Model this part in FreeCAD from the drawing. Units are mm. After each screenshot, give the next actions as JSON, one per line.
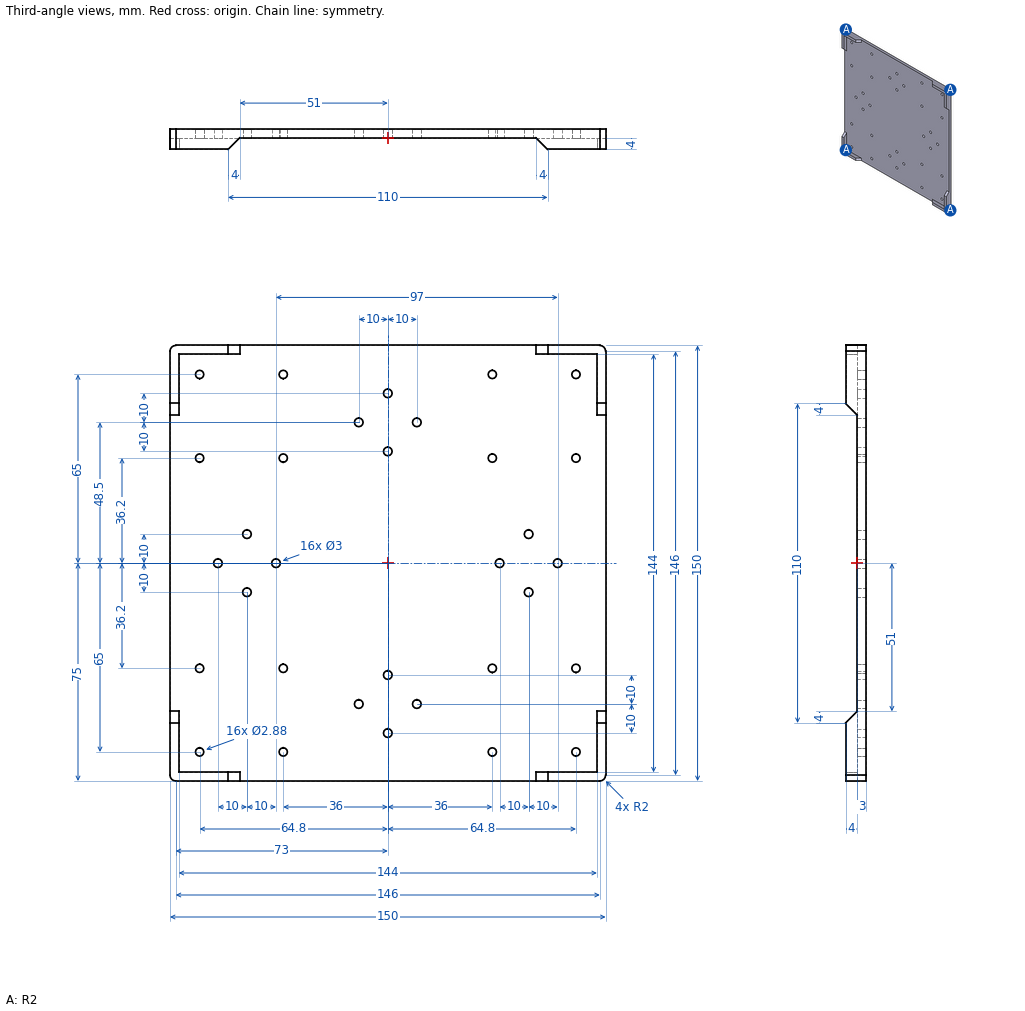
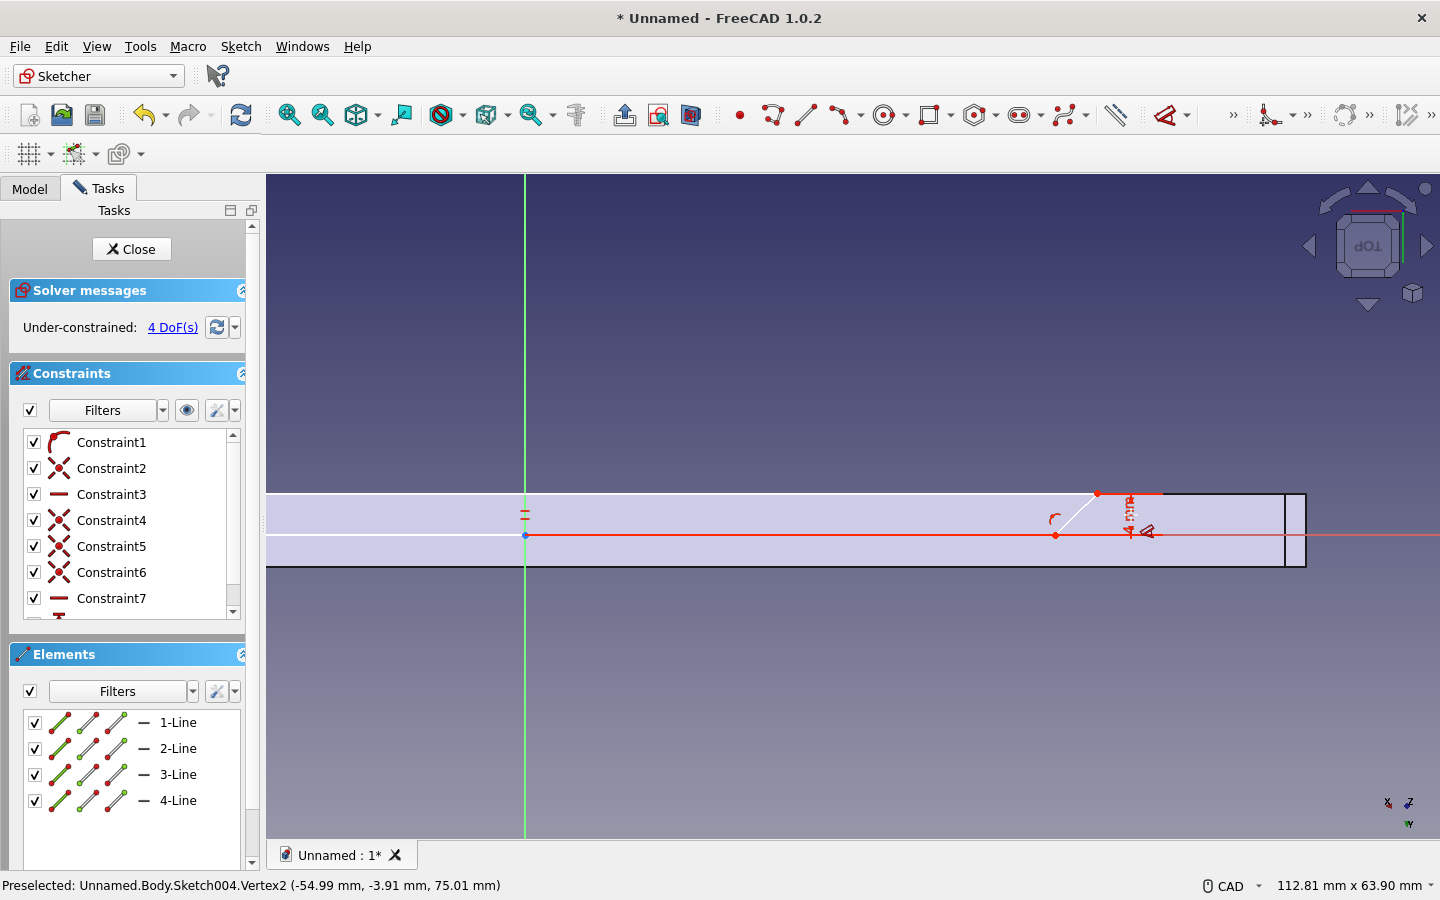
{"action": "left_click", "coordinate": [1068, 523]}
{"action": "left_click", "coordinate": [1076, 569]}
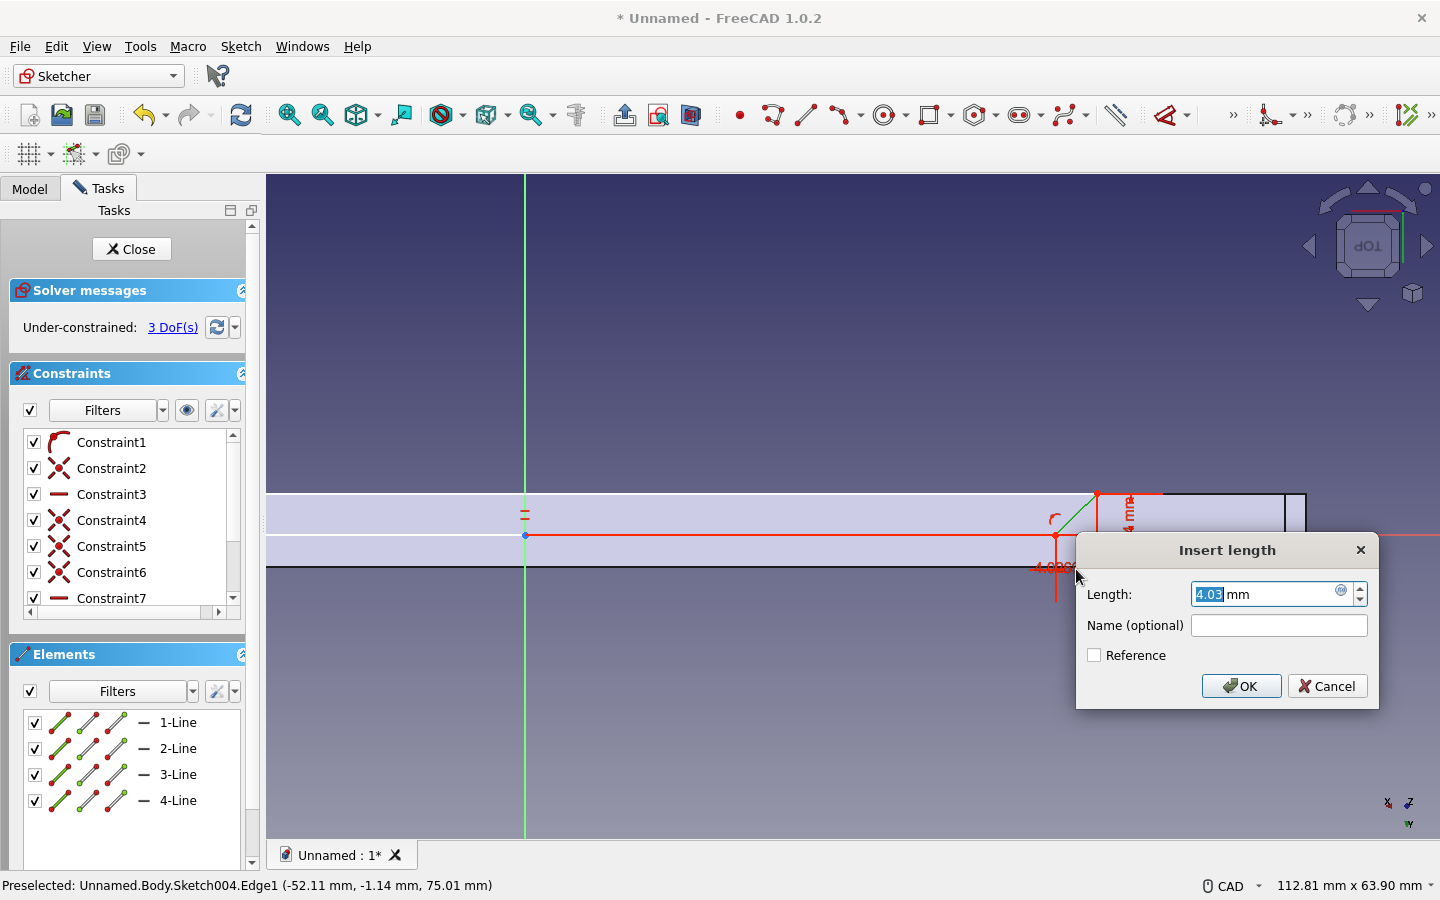
{"action": "type", "text": "4"}
{"action": "key", "text": "Return"}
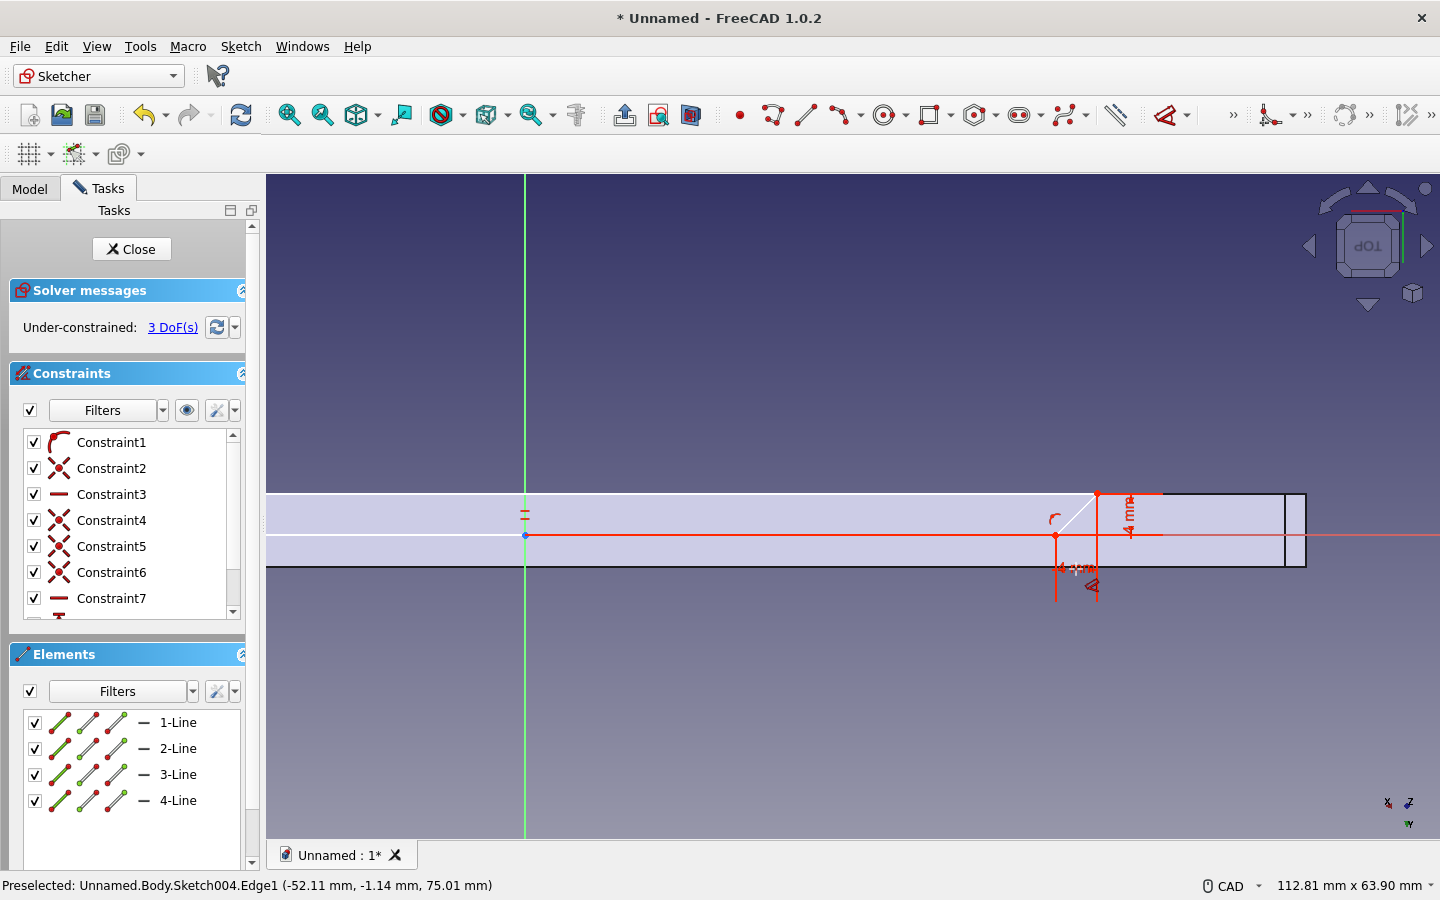
{"action": "scroll", "coordinate": [1100, 497], "scroll_direction": "down", "scroll_amount": 3}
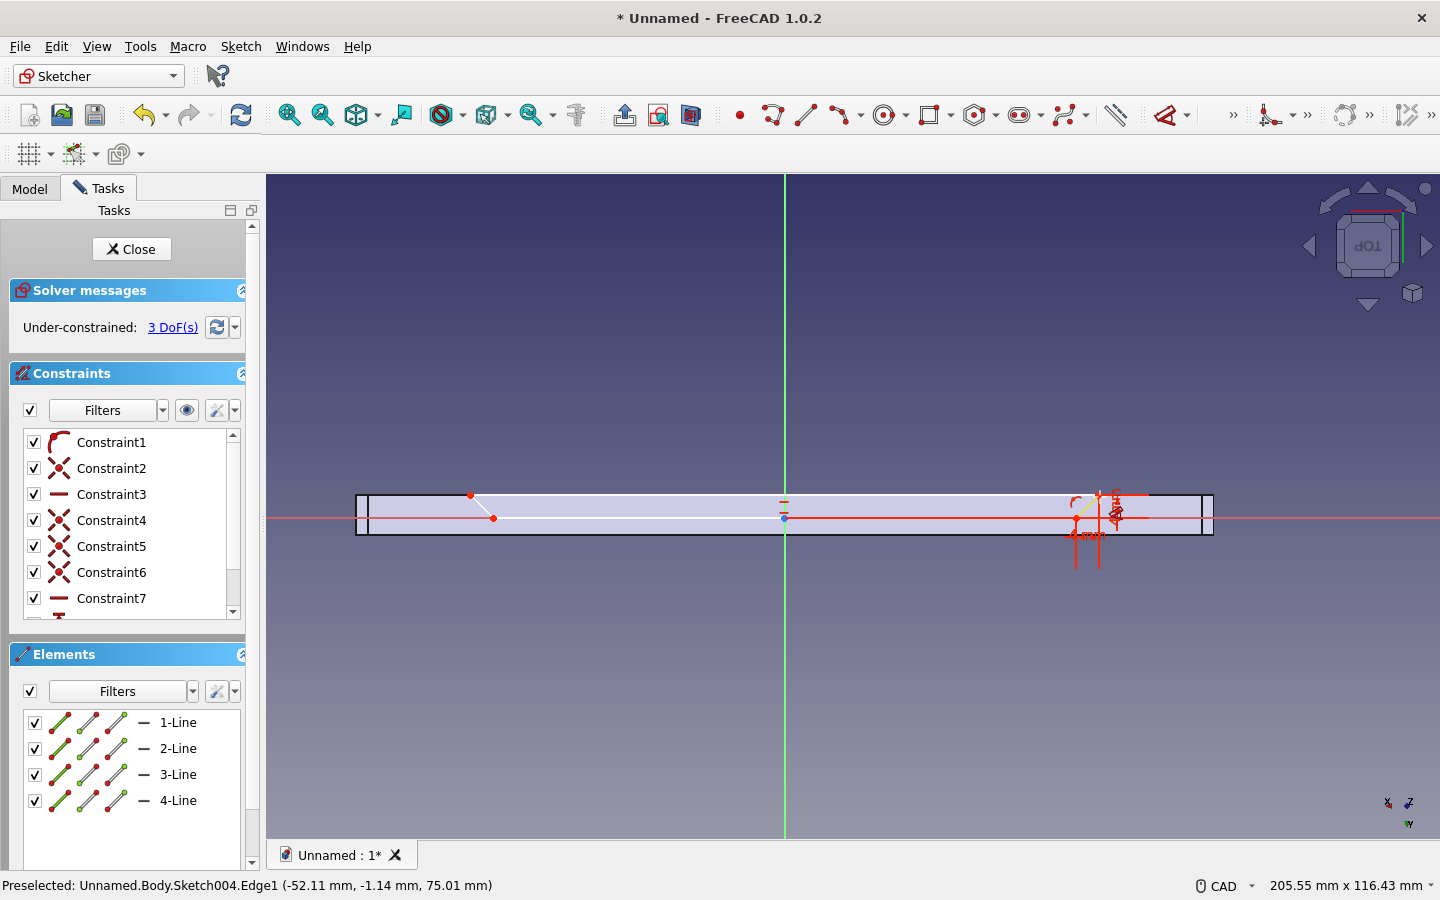
{"action": "scroll", "coordinate": [478, 502], "scroll_direction": "up", "scroll_amount": 4}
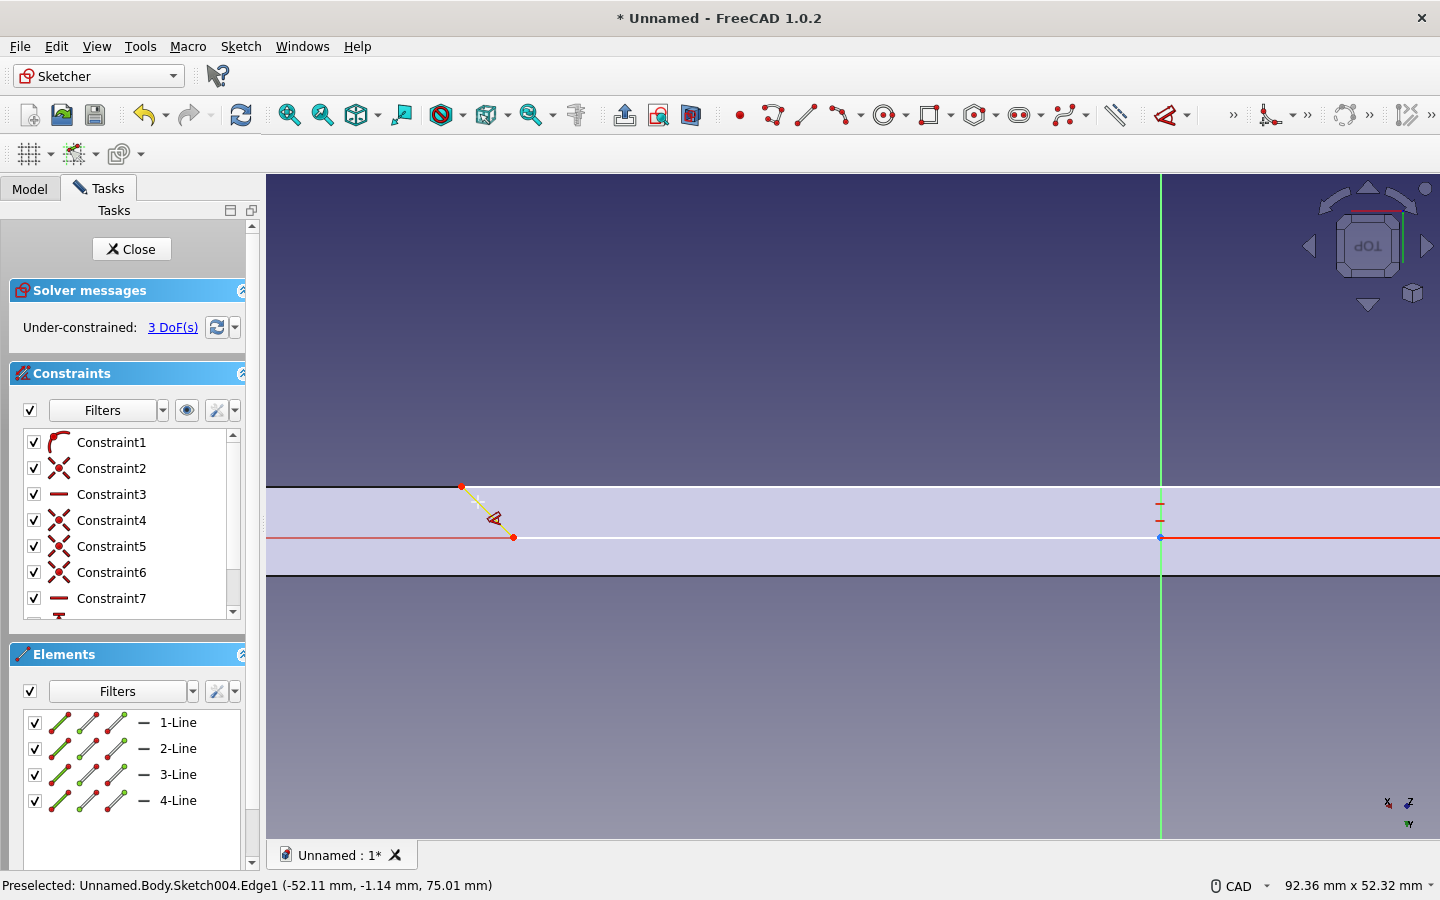
{"action": "left_click", "coordinate": [477, 502]}
{"action": "left_click", "coordinate": [488, 572]}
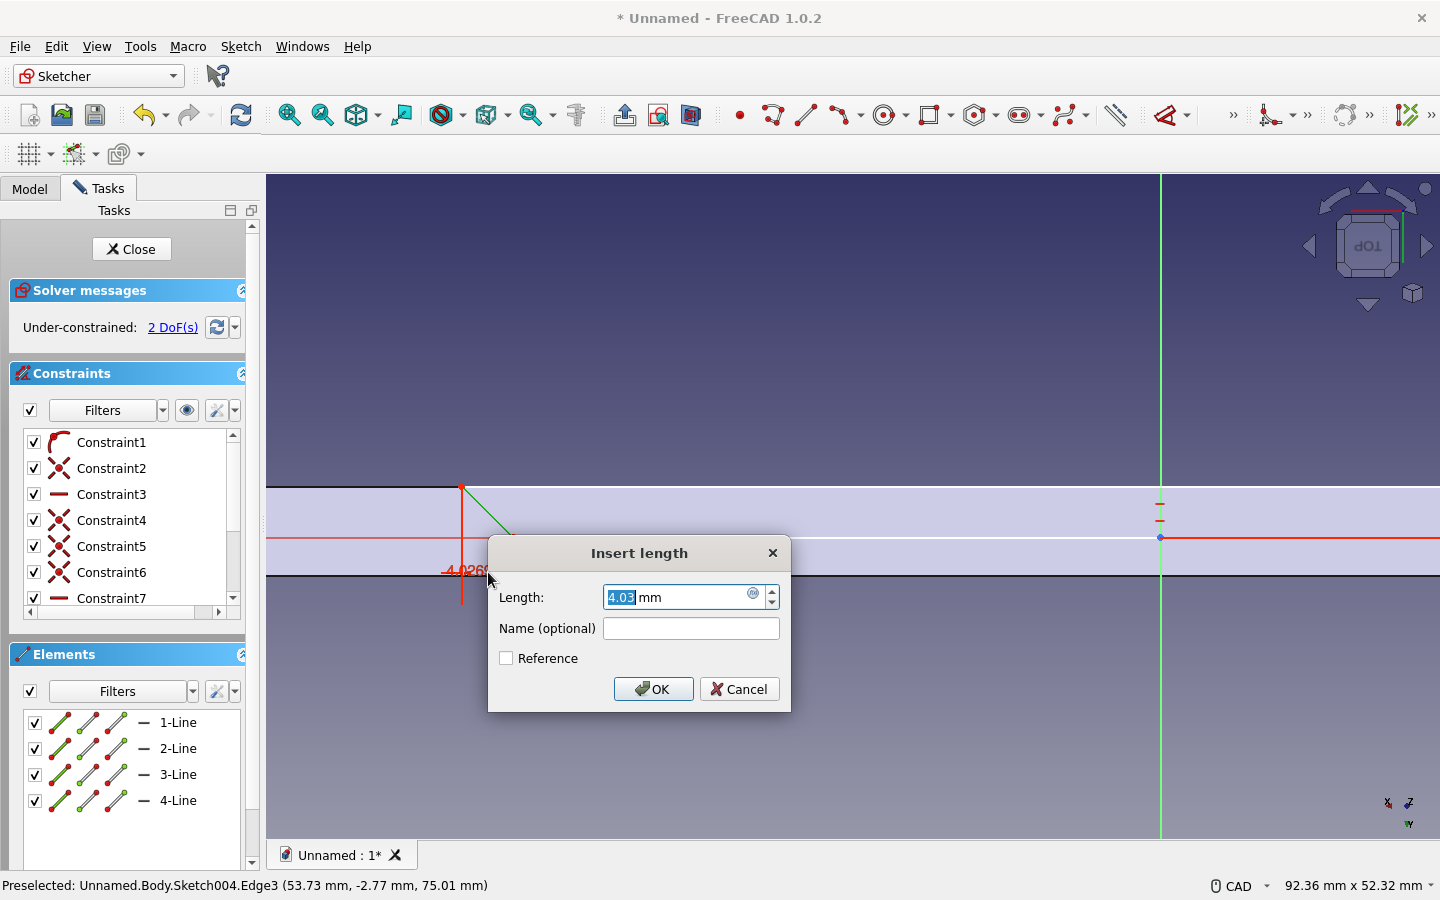
{"action": "type", "text": "4"}
{"action": "key", "text": "Return"}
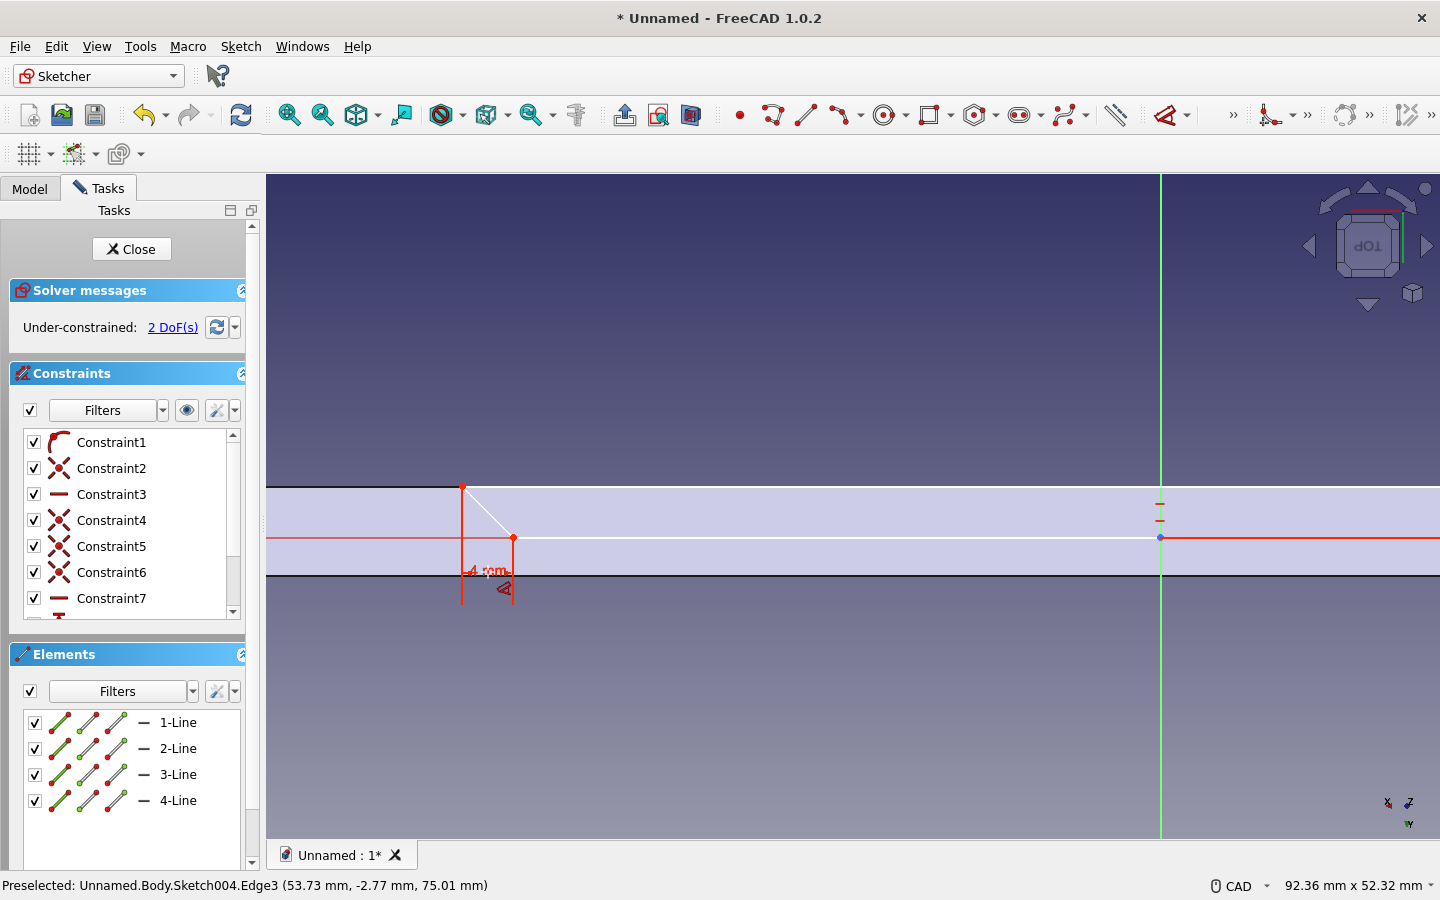
{"action": "left_click", "coordinate": [882, 487]}
{"action": "left_click", "coordinate": [869, 453]}